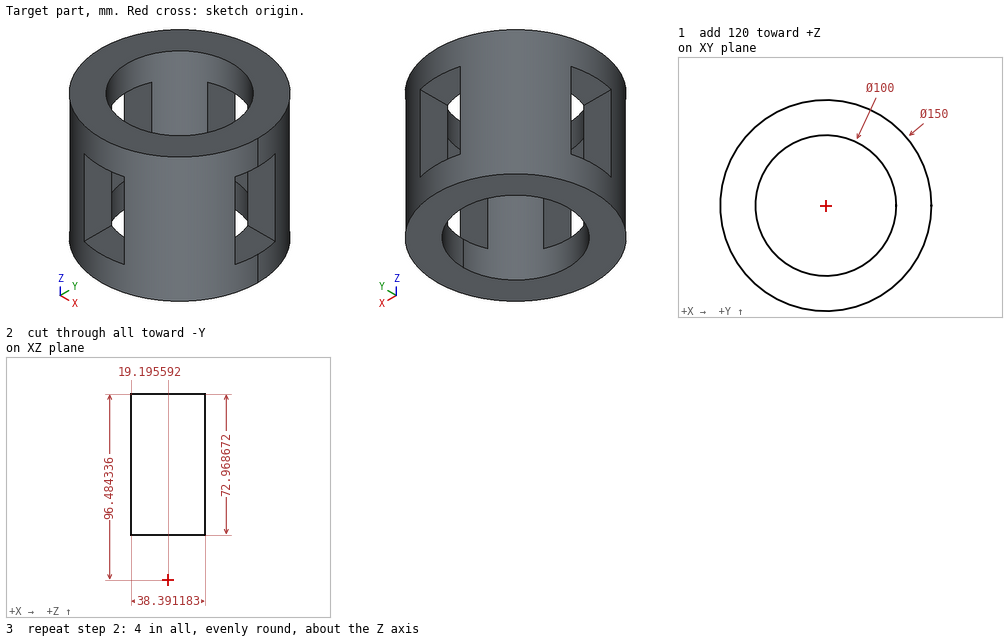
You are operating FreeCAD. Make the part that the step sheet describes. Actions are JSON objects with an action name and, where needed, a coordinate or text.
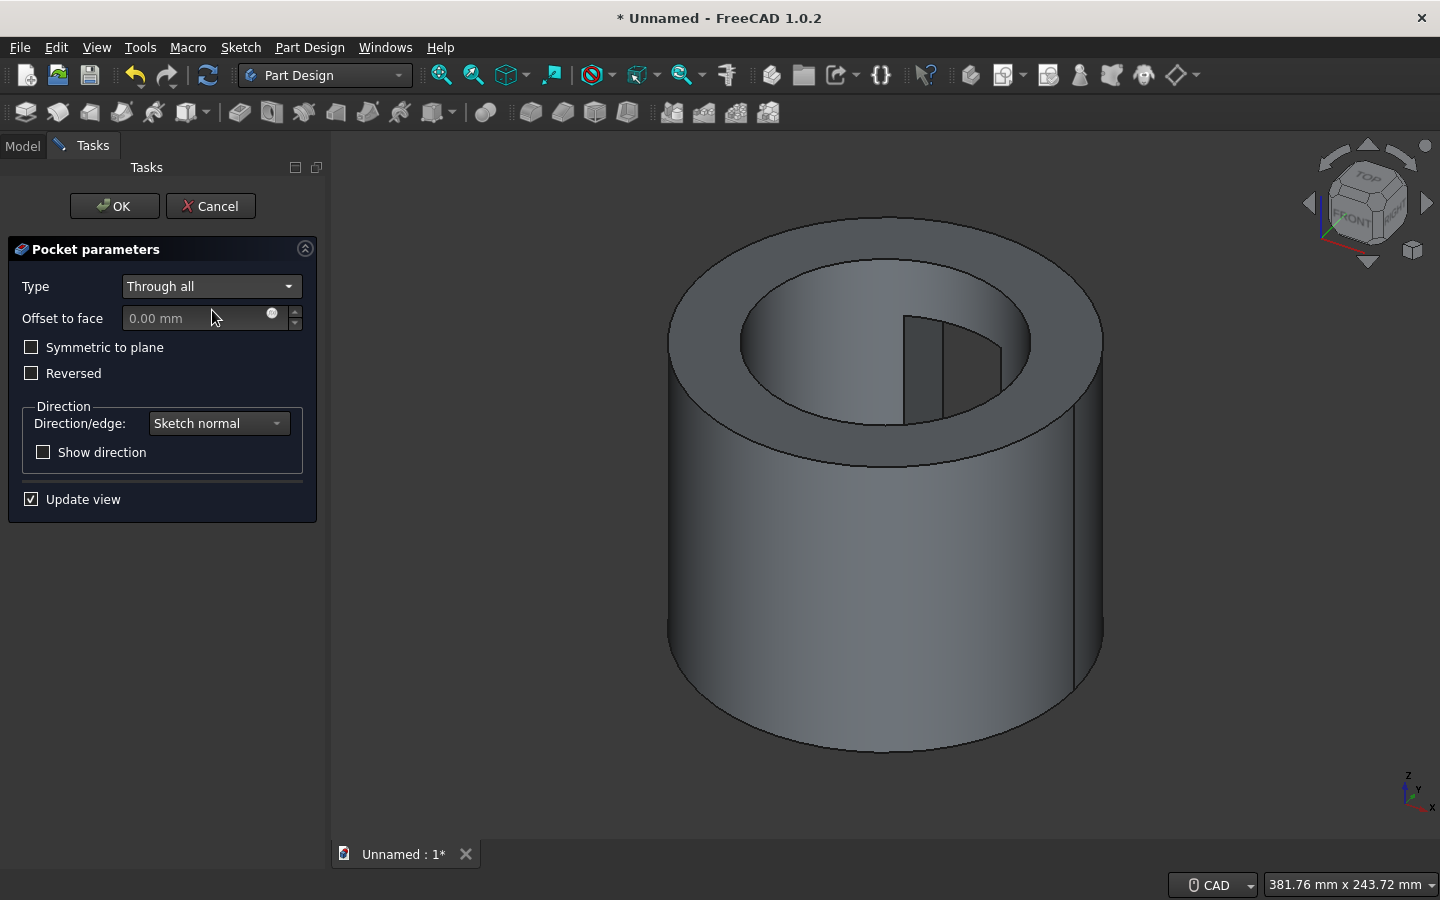
{"action": "left_click", "coordinate": [30, 373]}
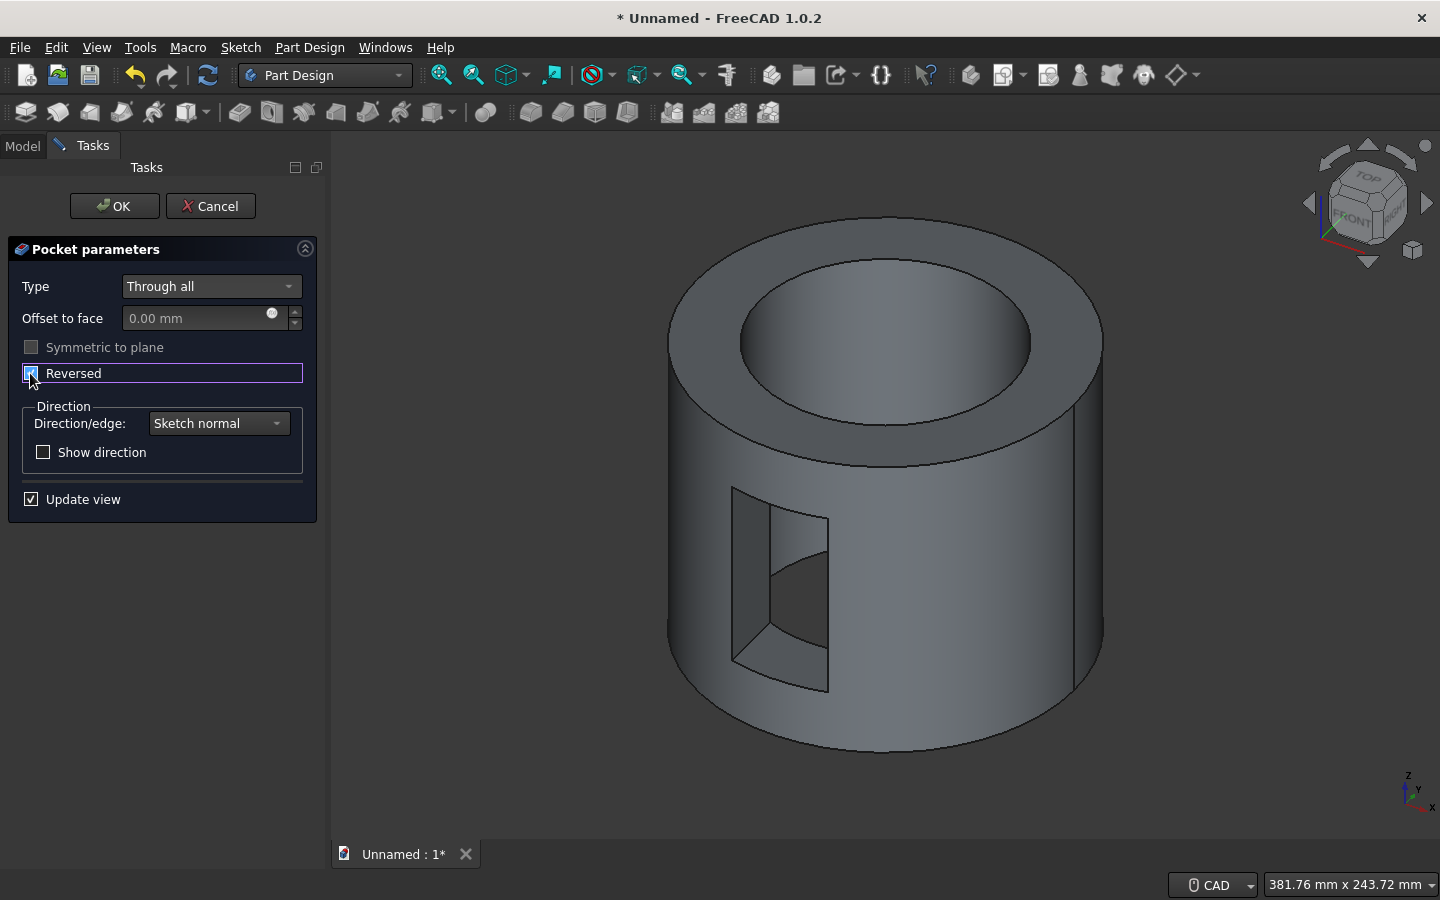
{"action": "left_click", "coordinate": [115, 206]}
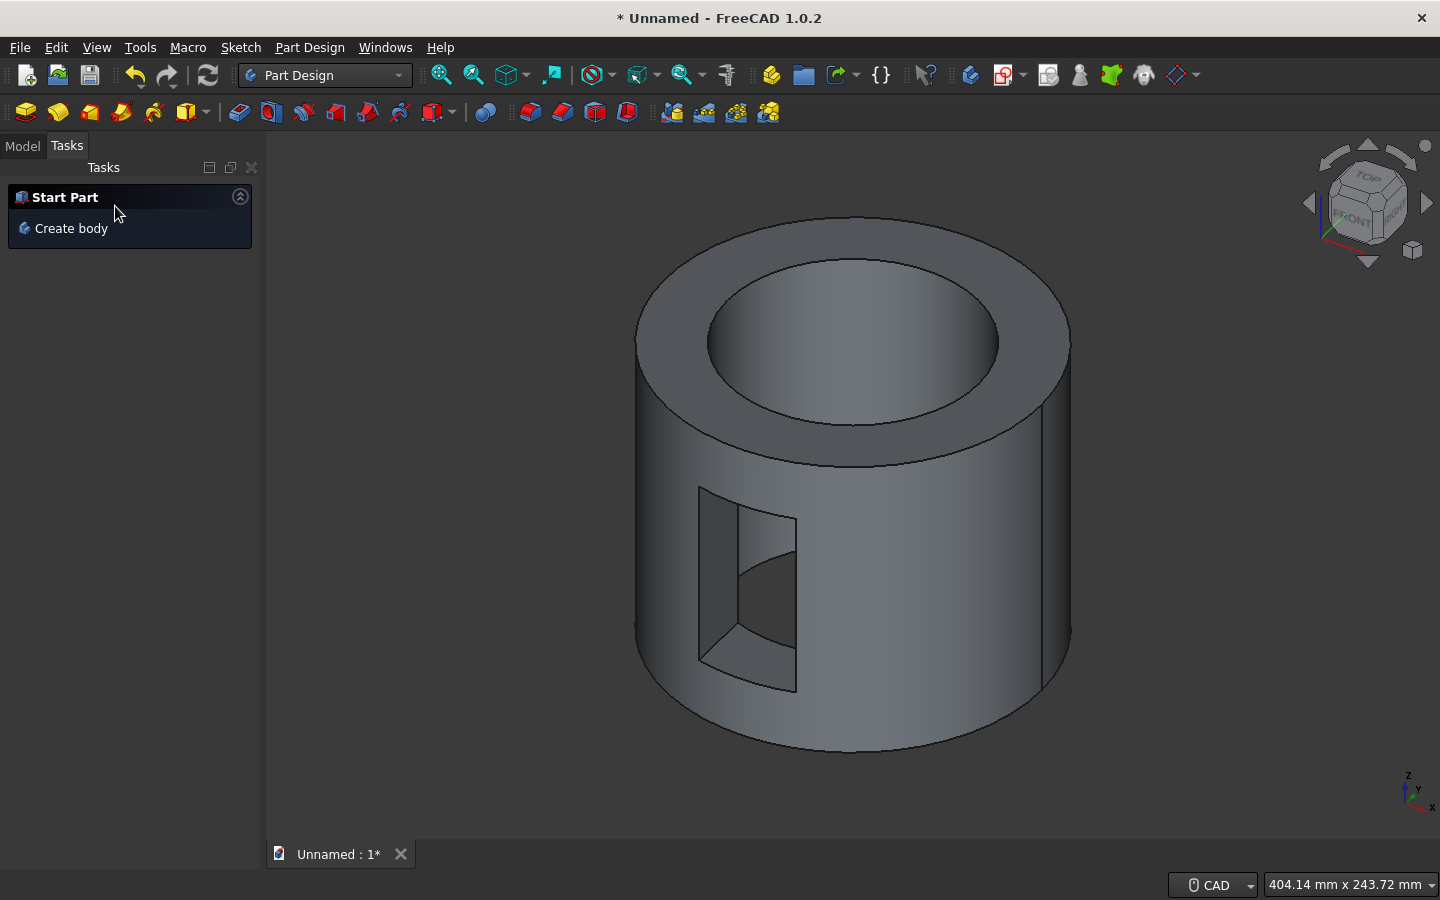
{"action": "left_click", "coordinate": [23, 145]}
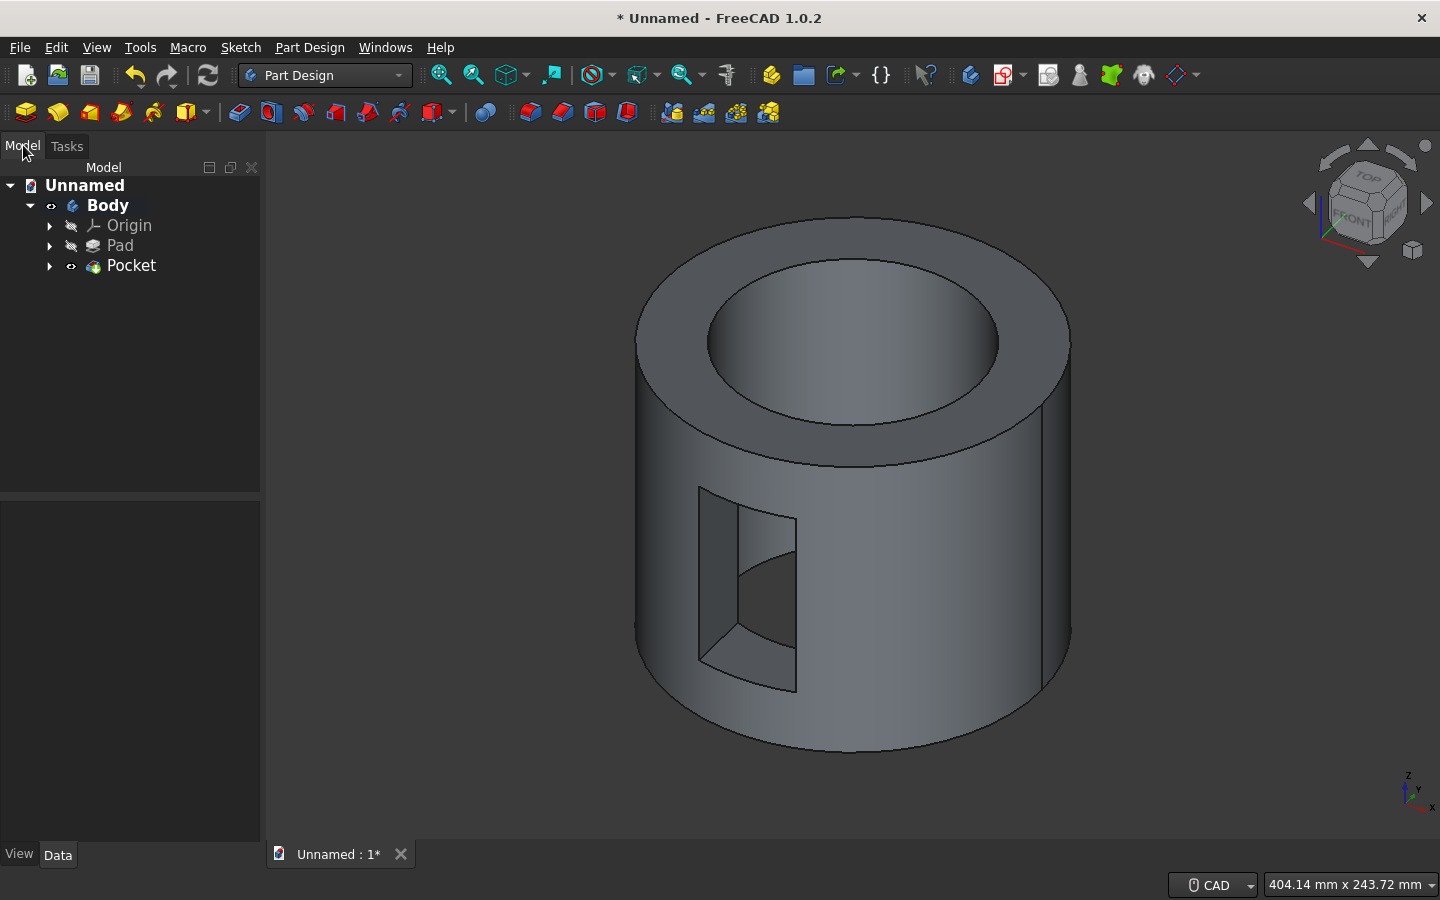
{"action": "left_click", "coordinate": [116, 266]}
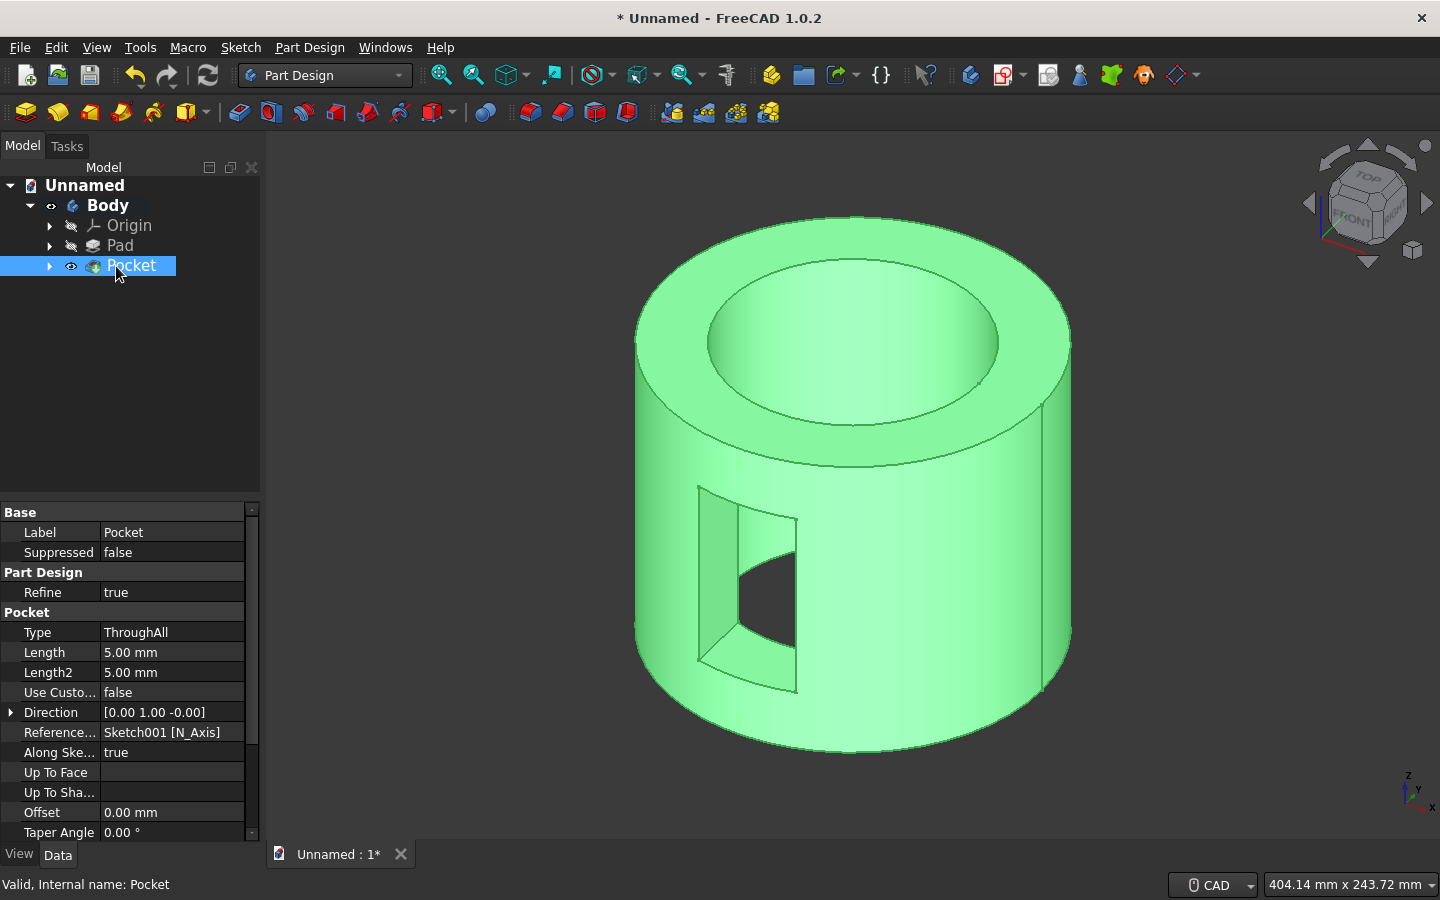
{"action": "left_click", "coordinate": [736, 112]}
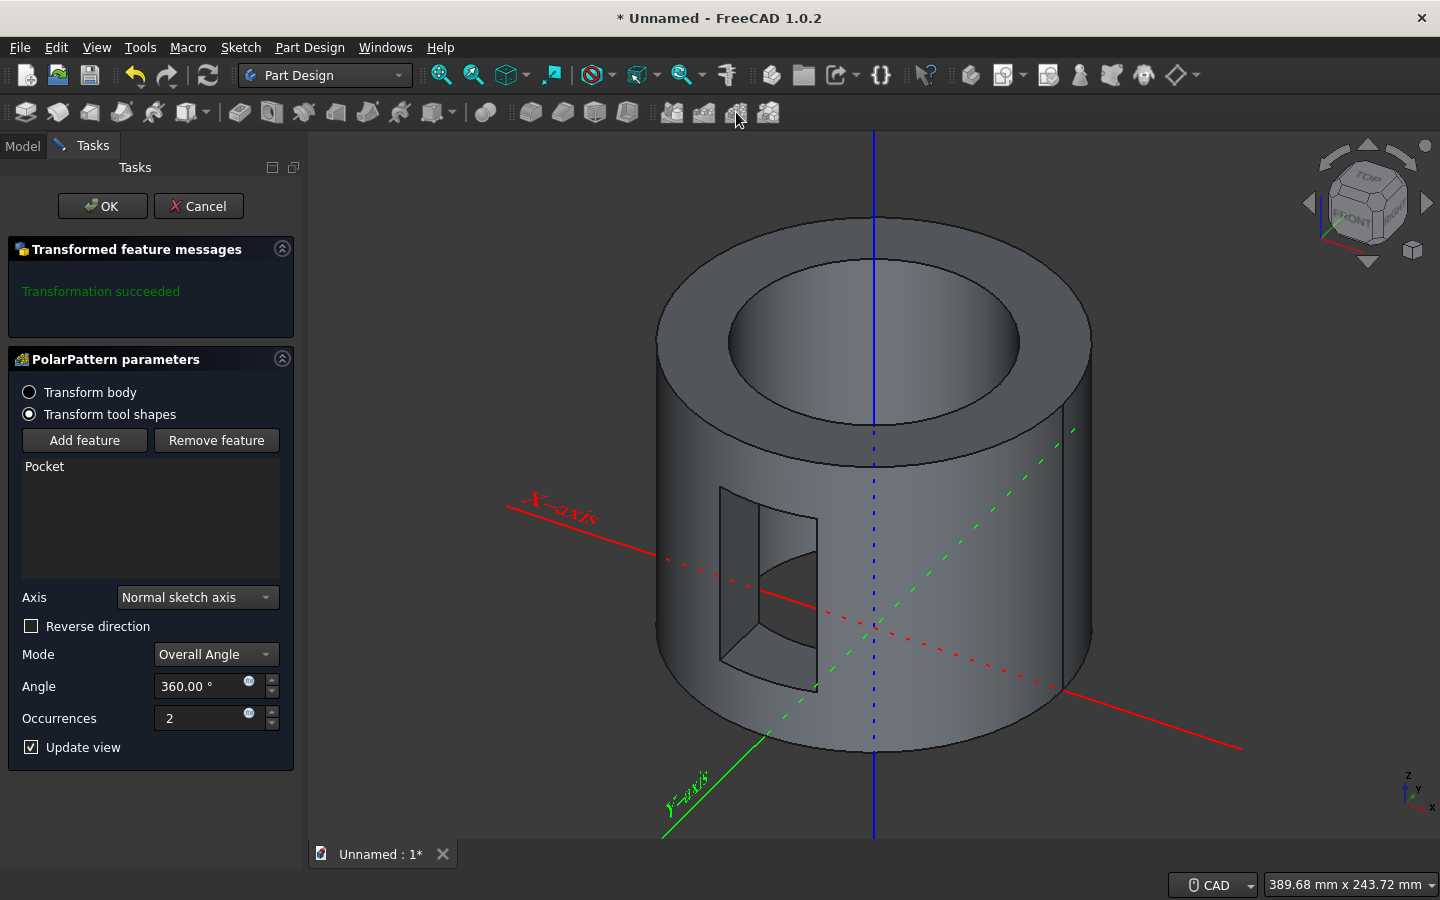
{"action": "left_click", "coordinate": [198, 598]}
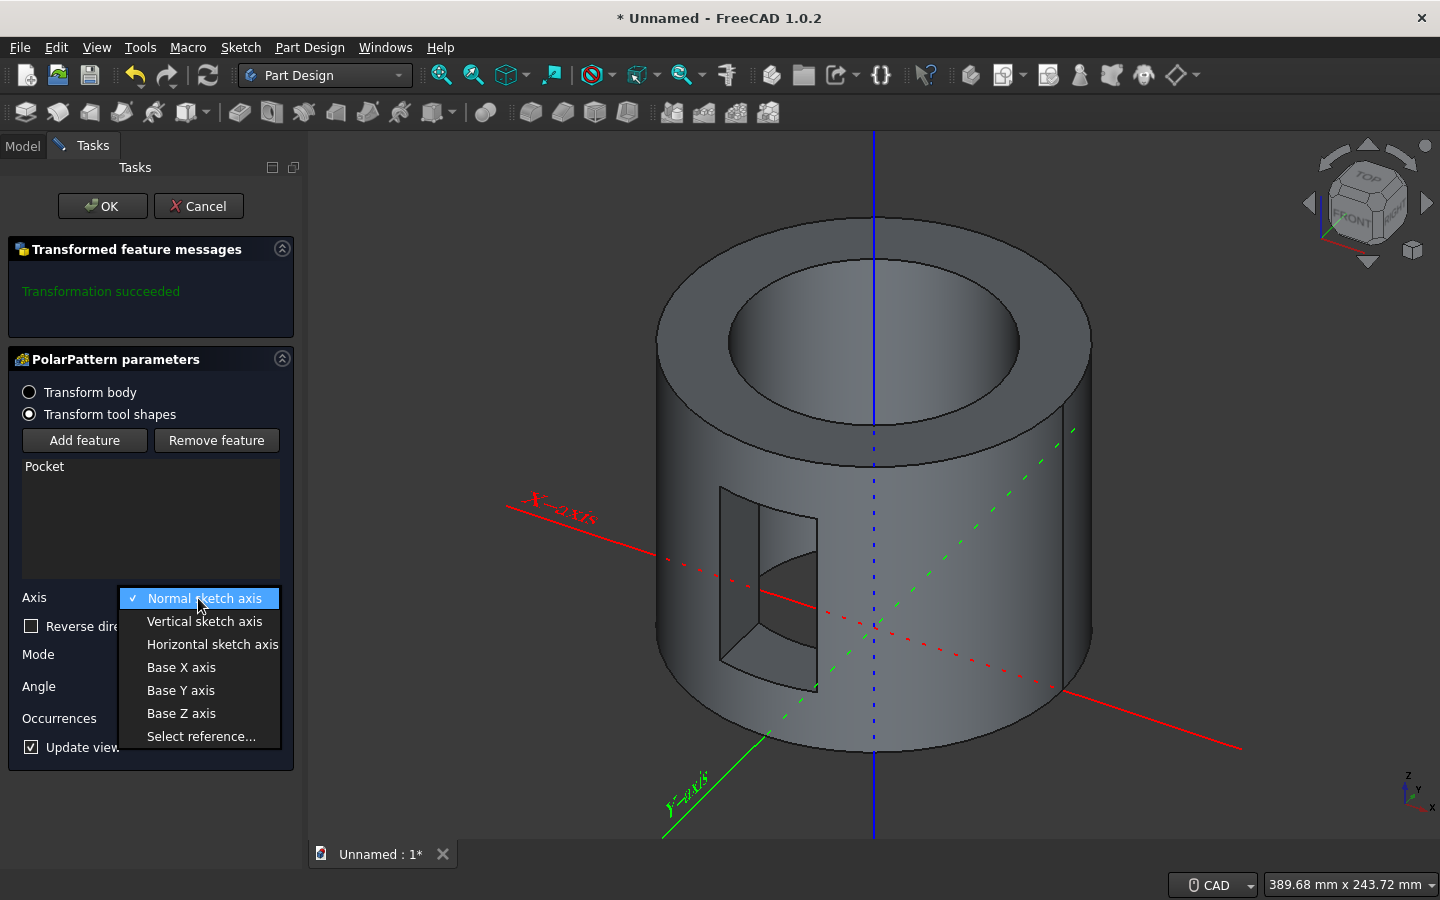
{"action": "left_click", "coordinate": [198, 714]}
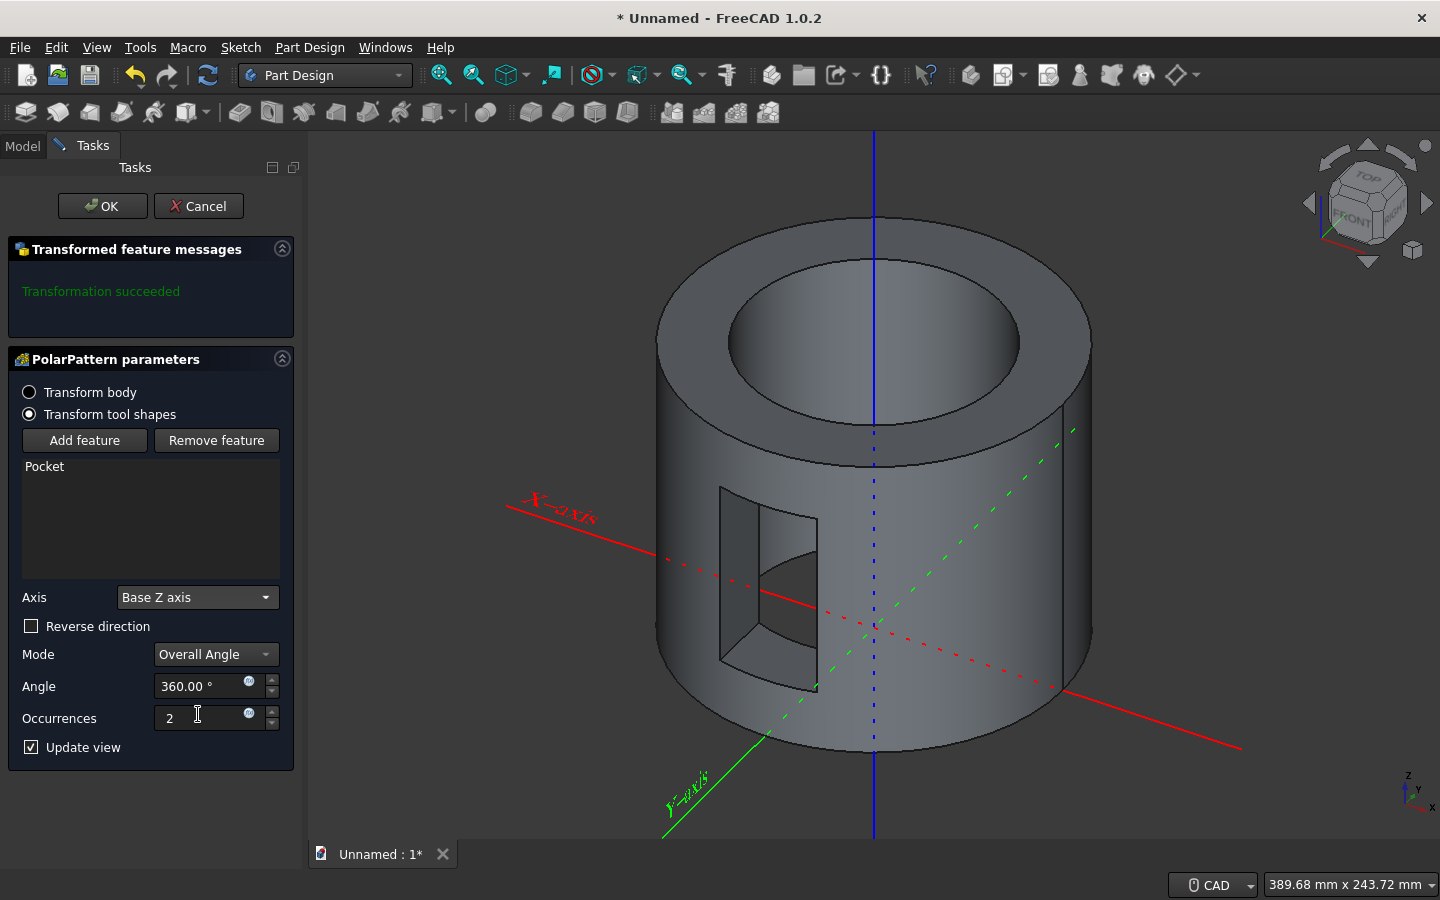
{"action": "triple_click", "coordinate": [209, 718]}